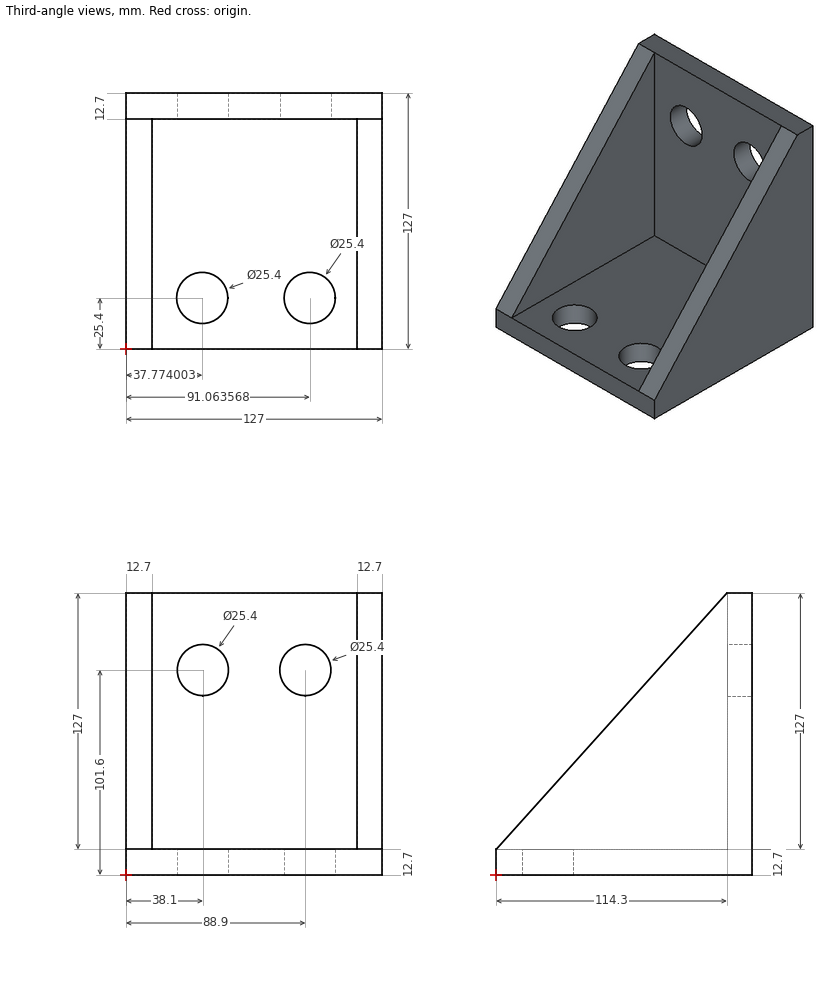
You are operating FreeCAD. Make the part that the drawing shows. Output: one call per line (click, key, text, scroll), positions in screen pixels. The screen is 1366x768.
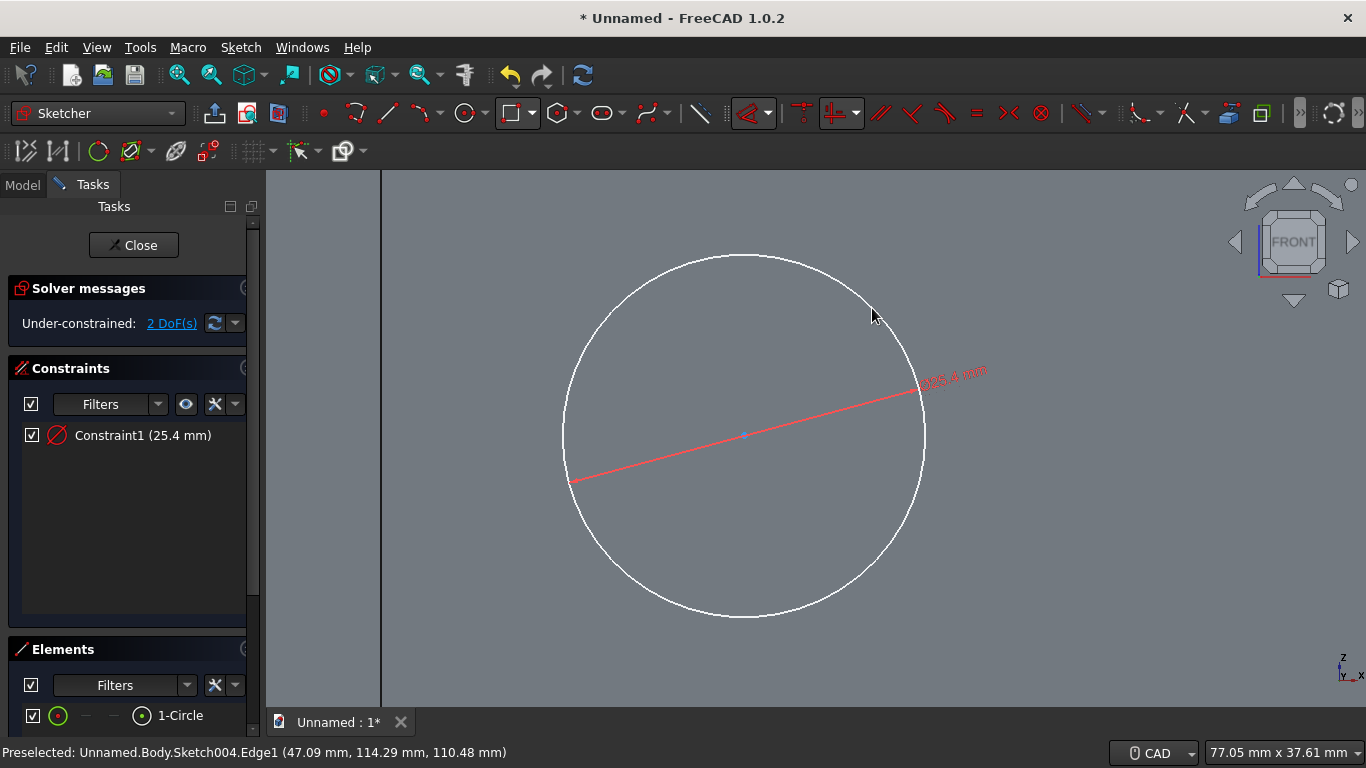
click(744, 436)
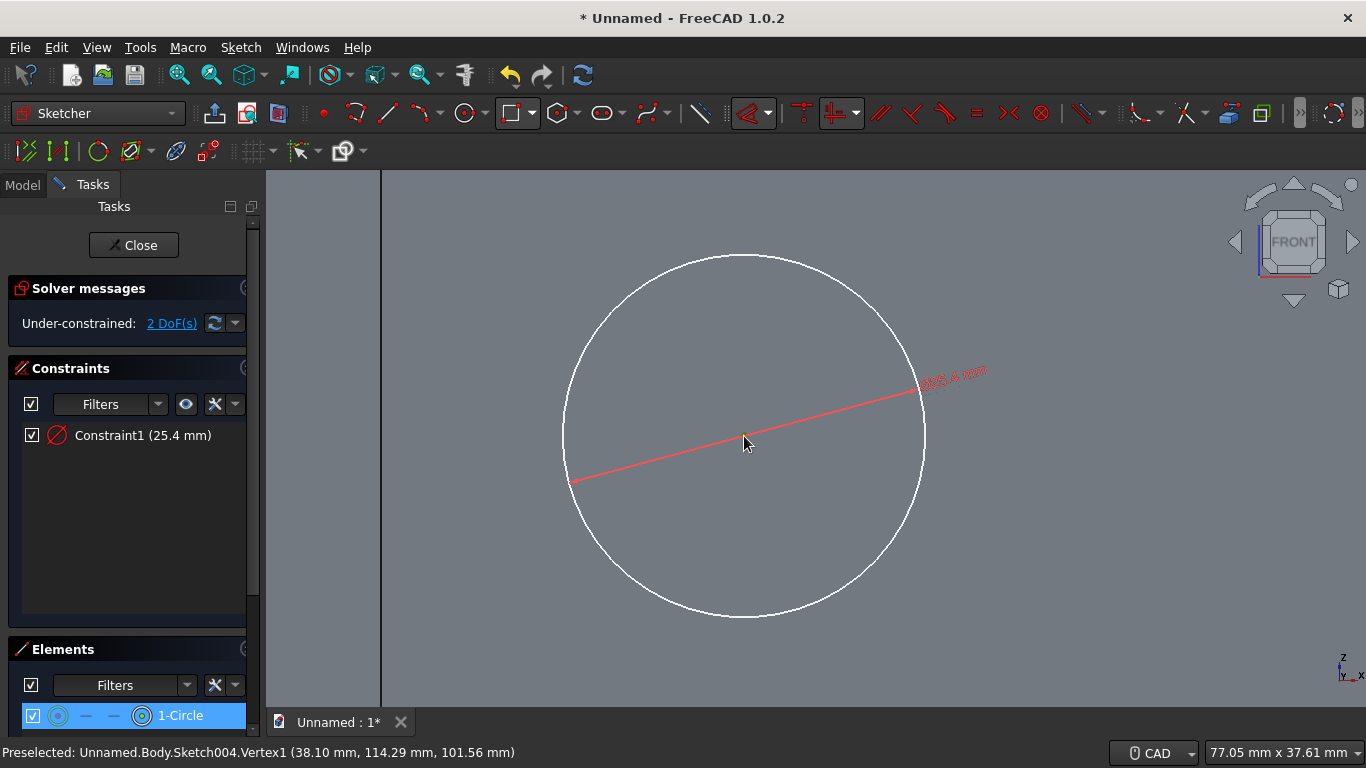
key(l)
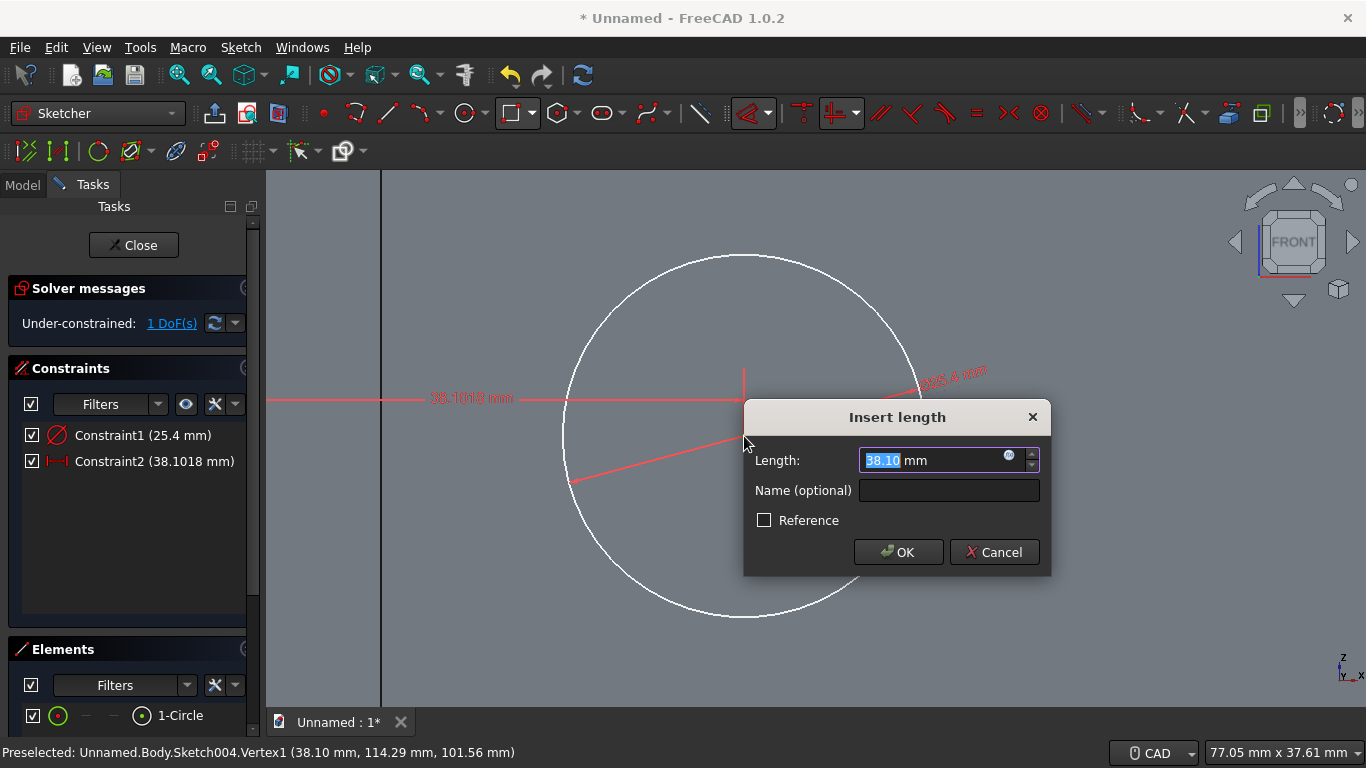
text(38.1)
key(Return)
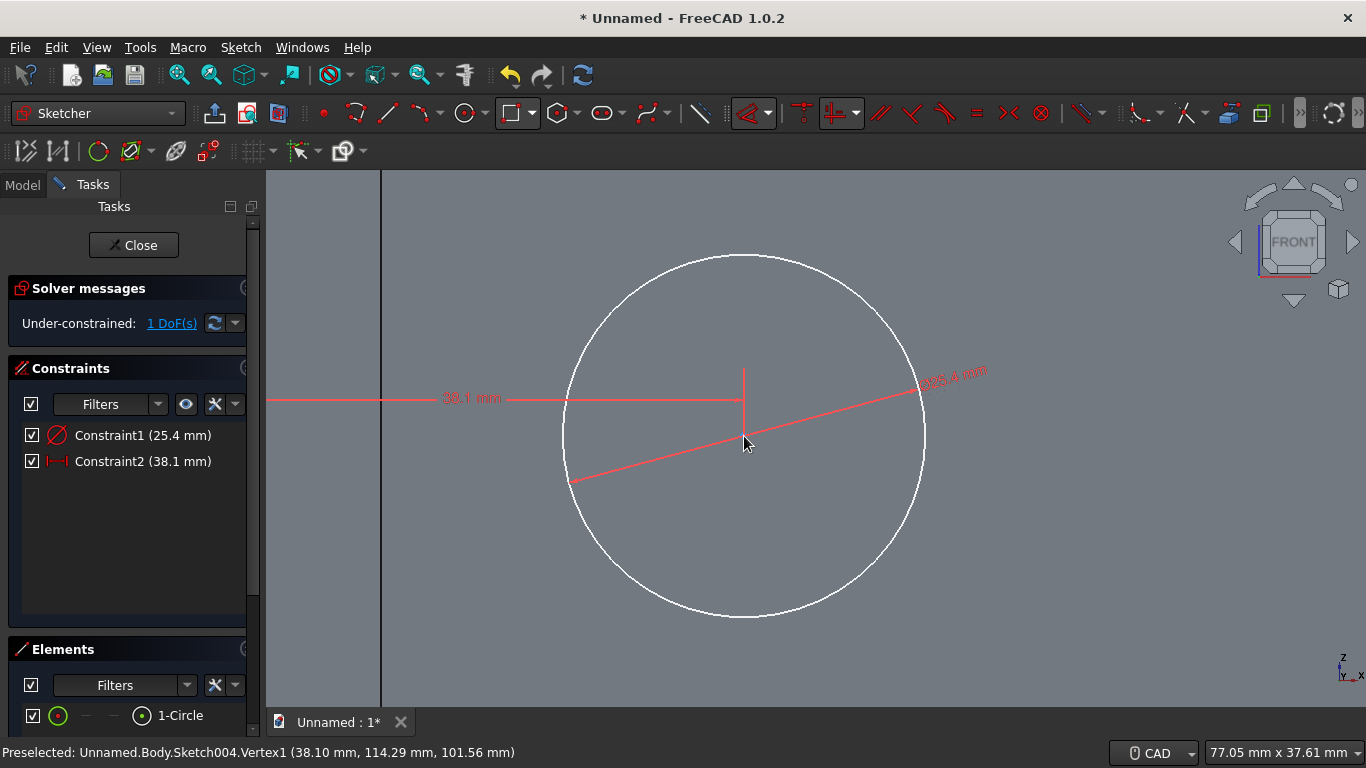
click(744, 436)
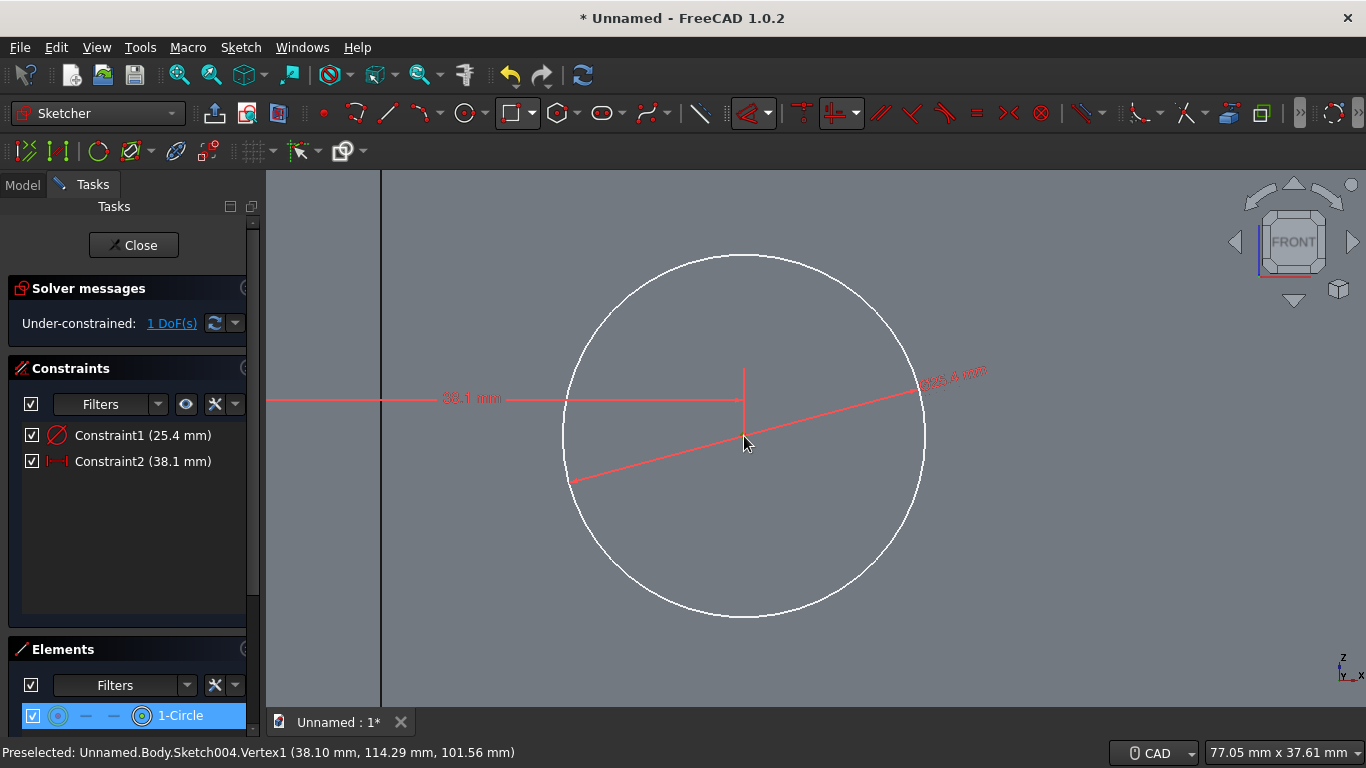
key(i)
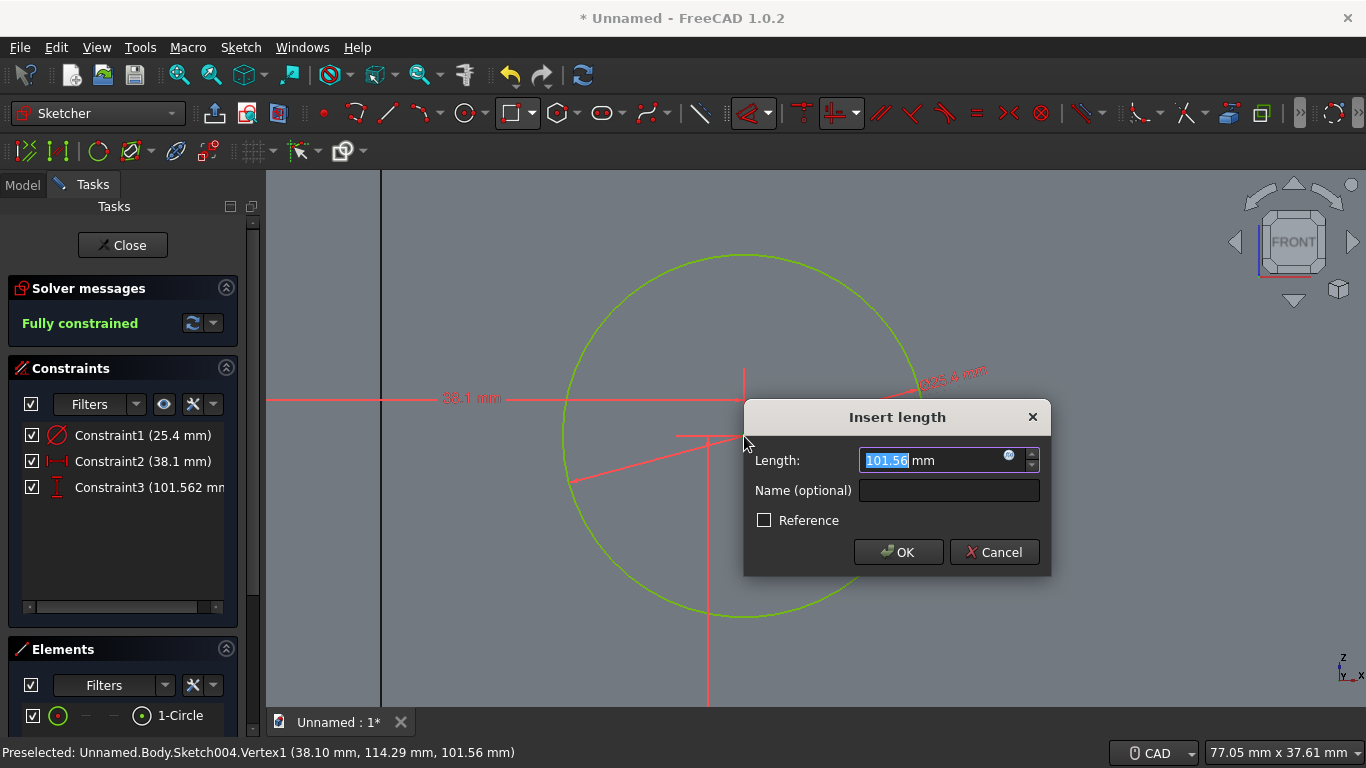
text(101.6)
key(Return)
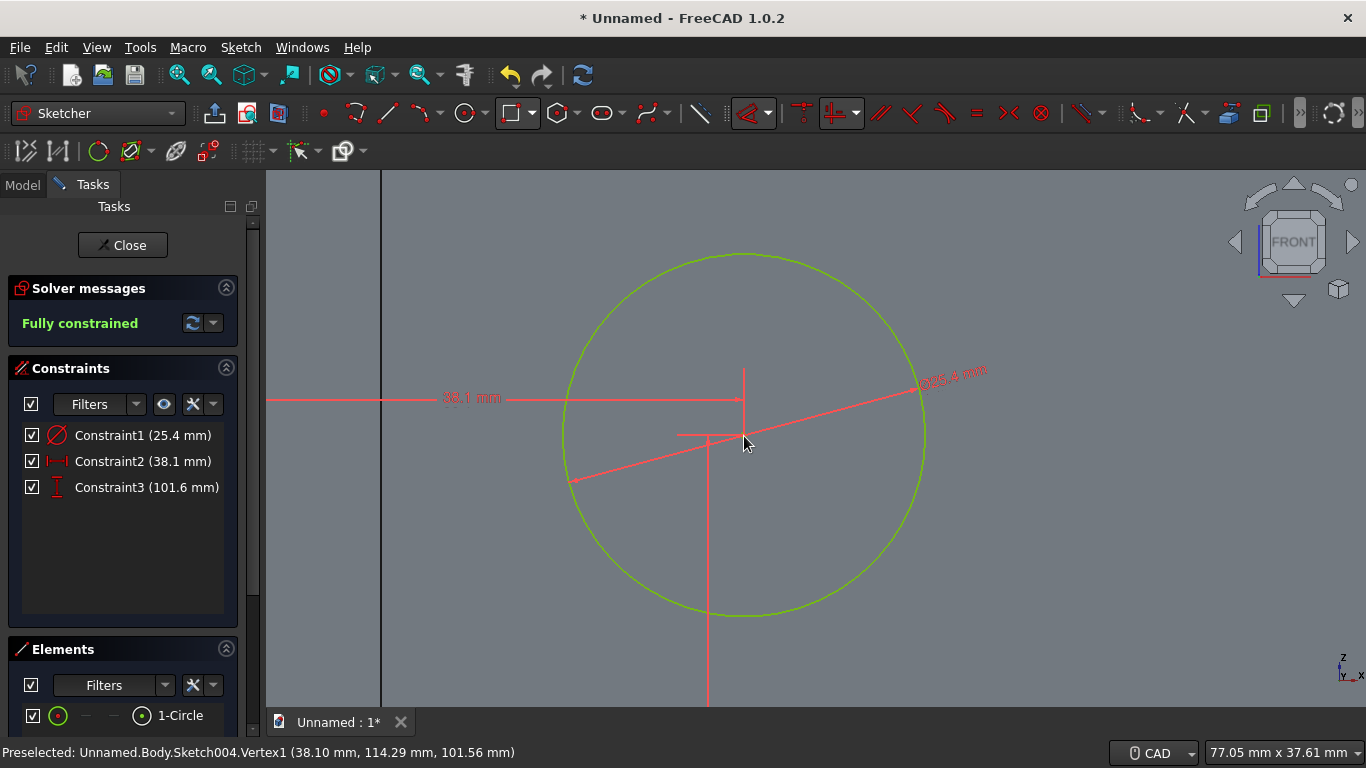
click(123, 245)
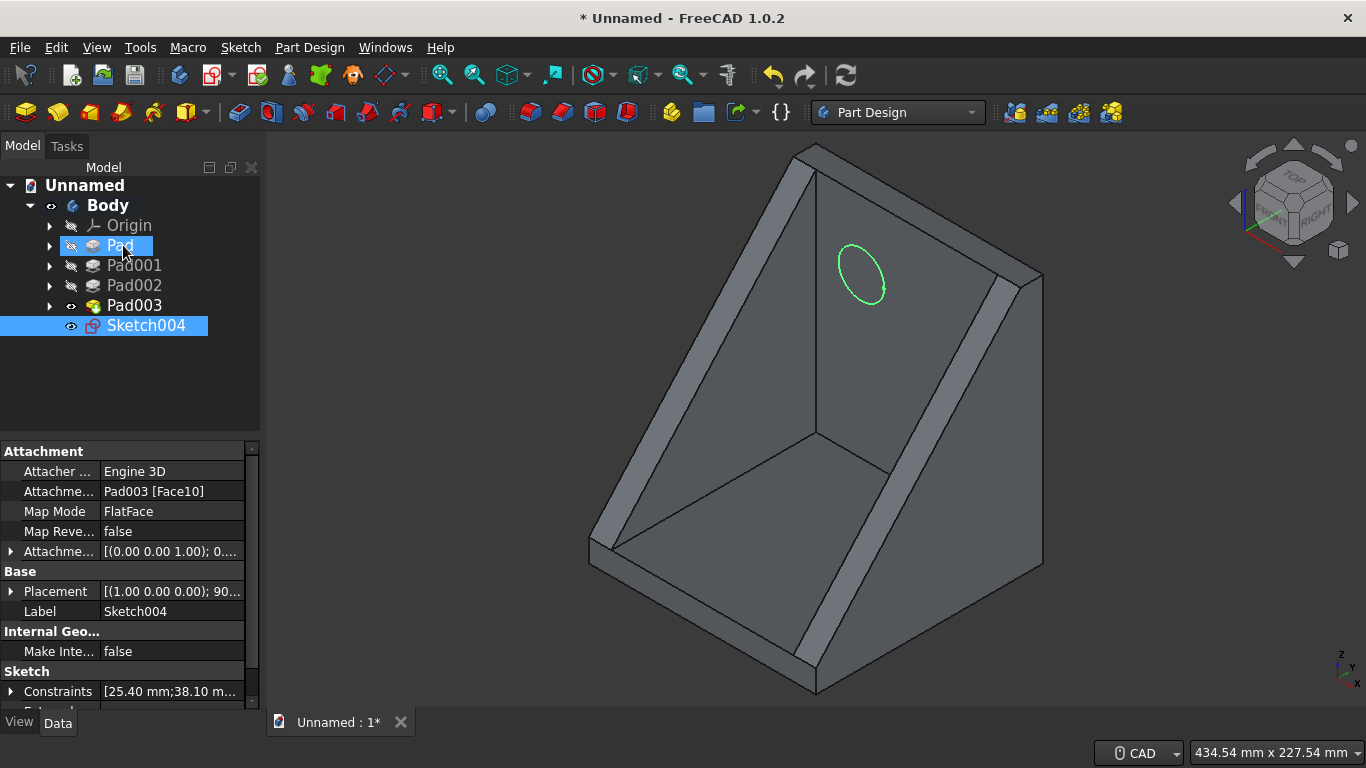
click(240, 112)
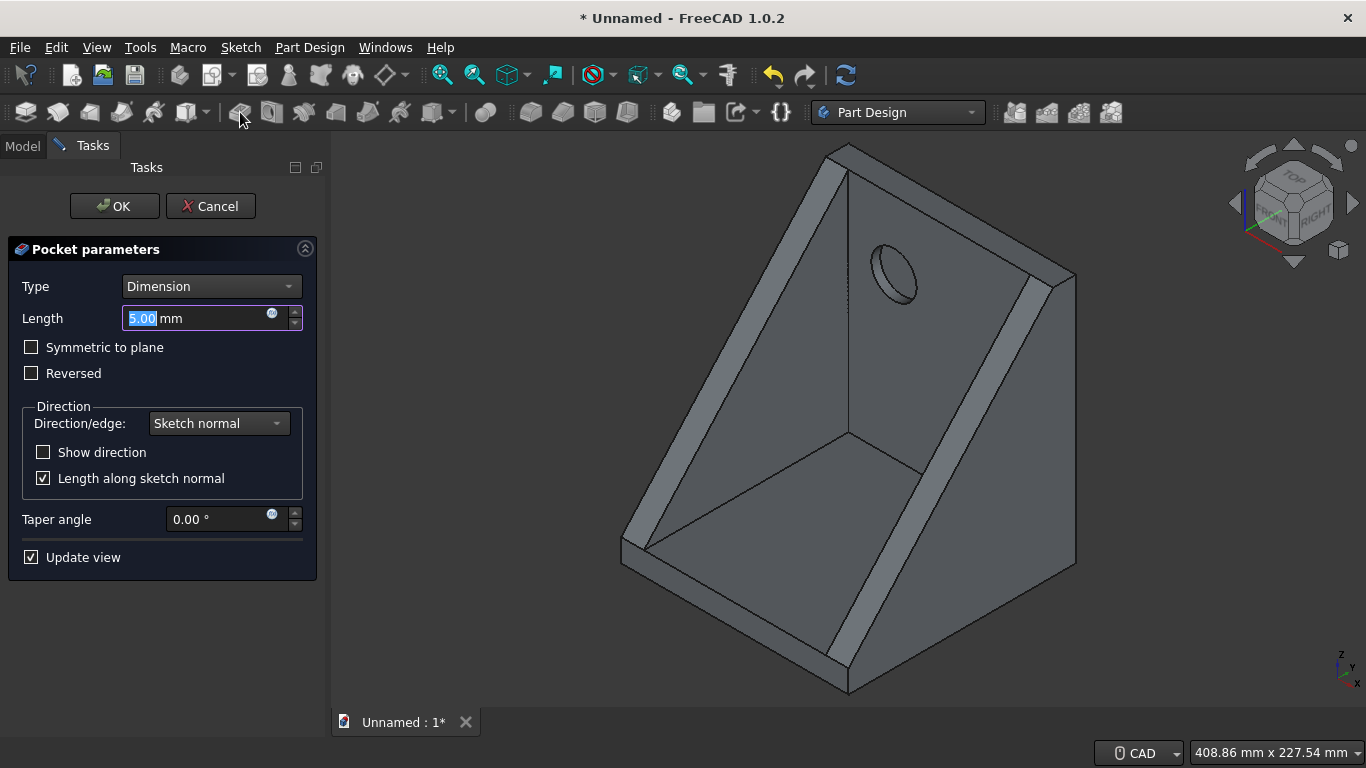
text(12.7)
key(Tab)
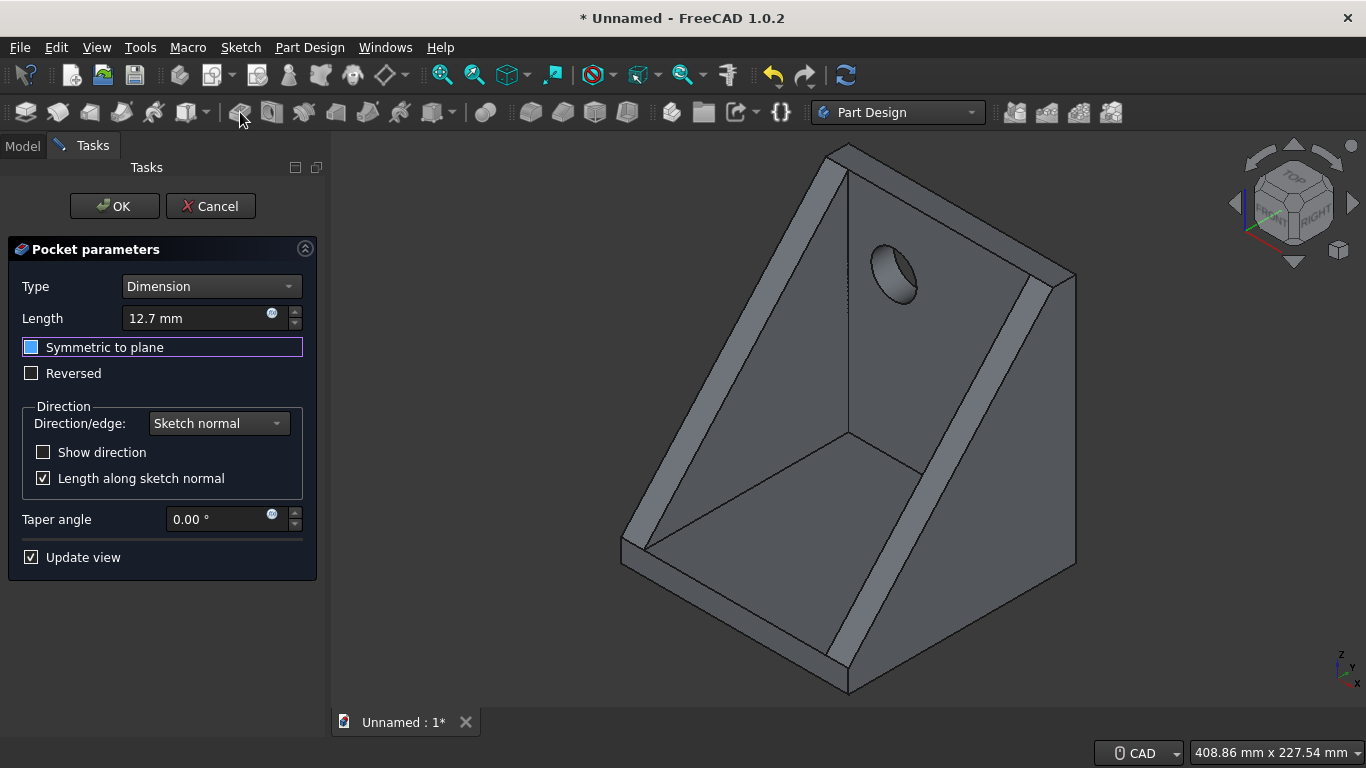
click(115, 206)